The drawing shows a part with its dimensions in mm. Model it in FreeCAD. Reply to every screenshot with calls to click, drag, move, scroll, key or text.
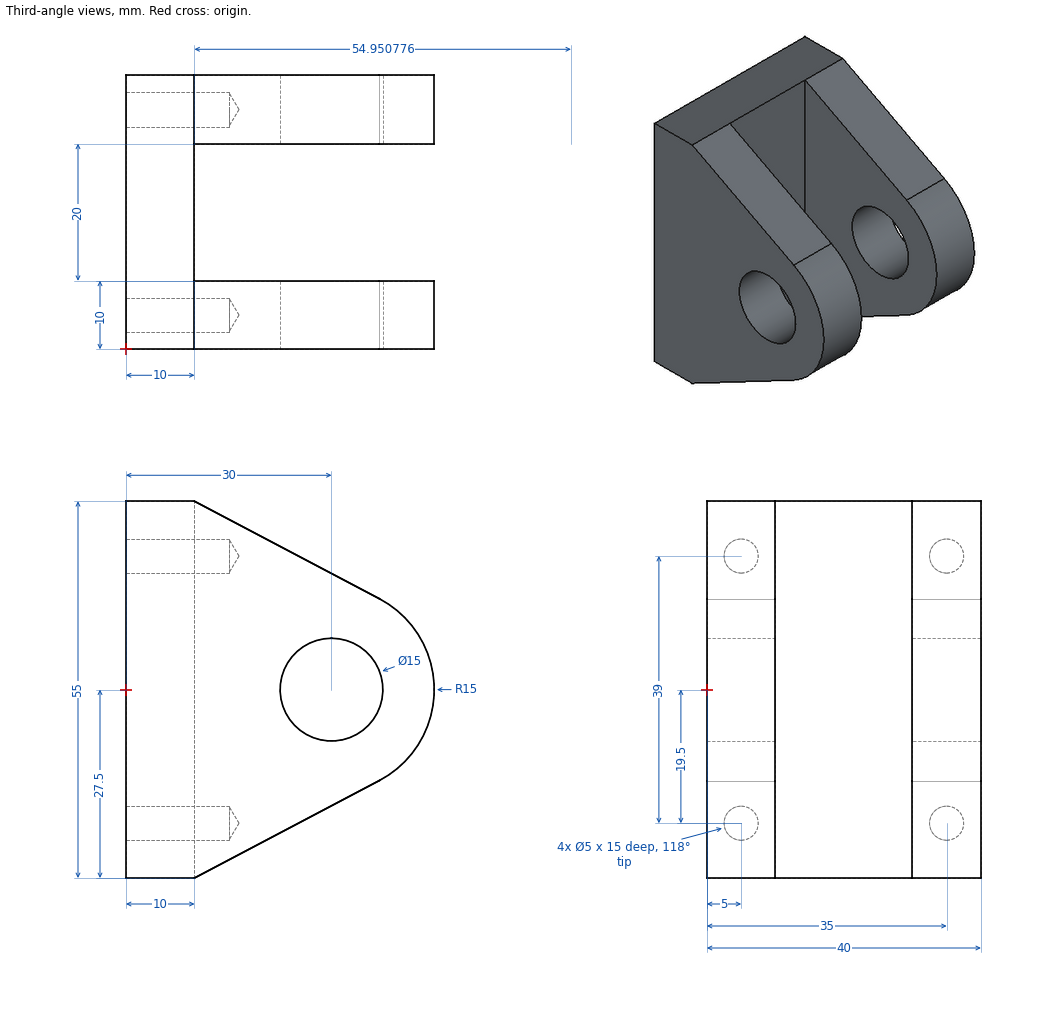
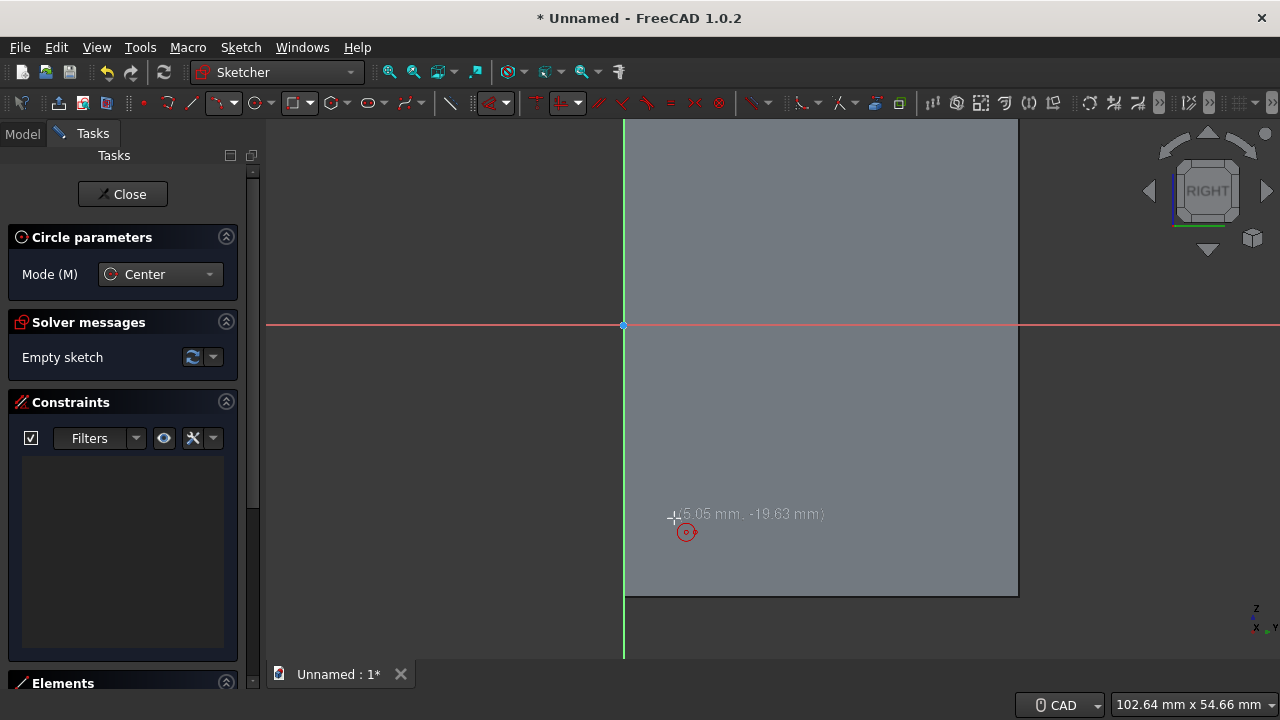
click(673, 518)
click(691, 500)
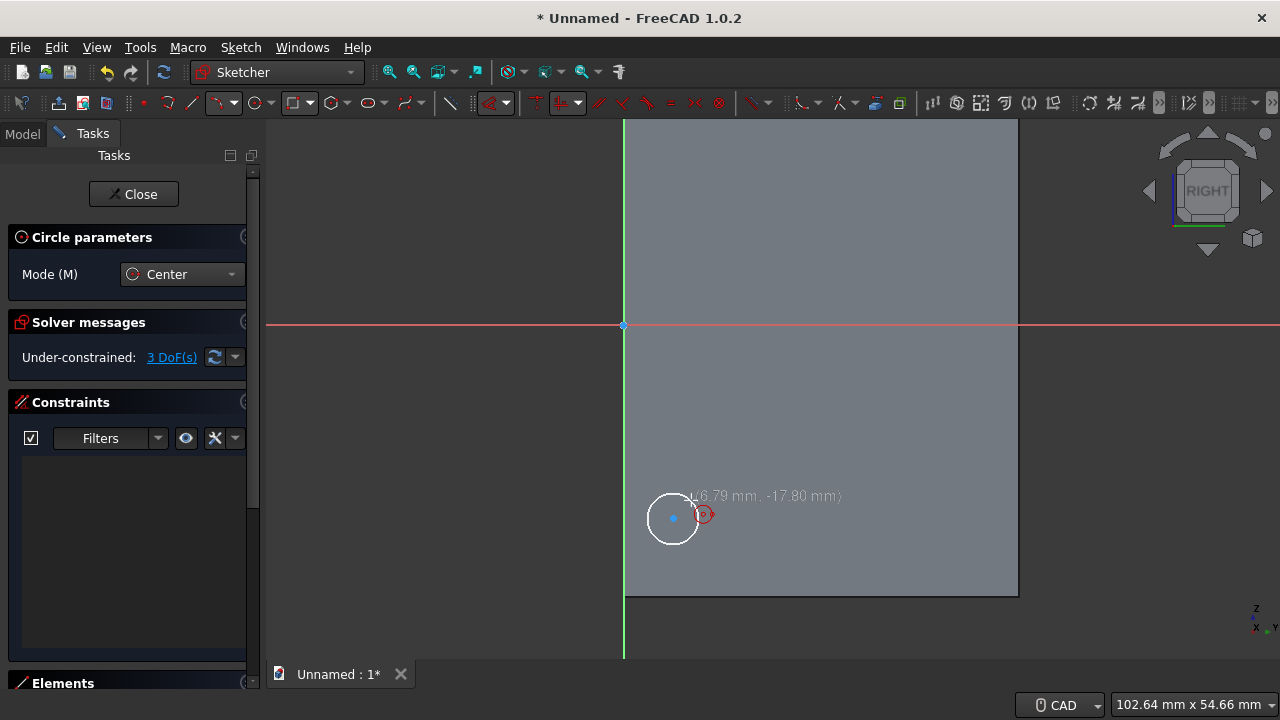
click(970, 518)
click(987, 500)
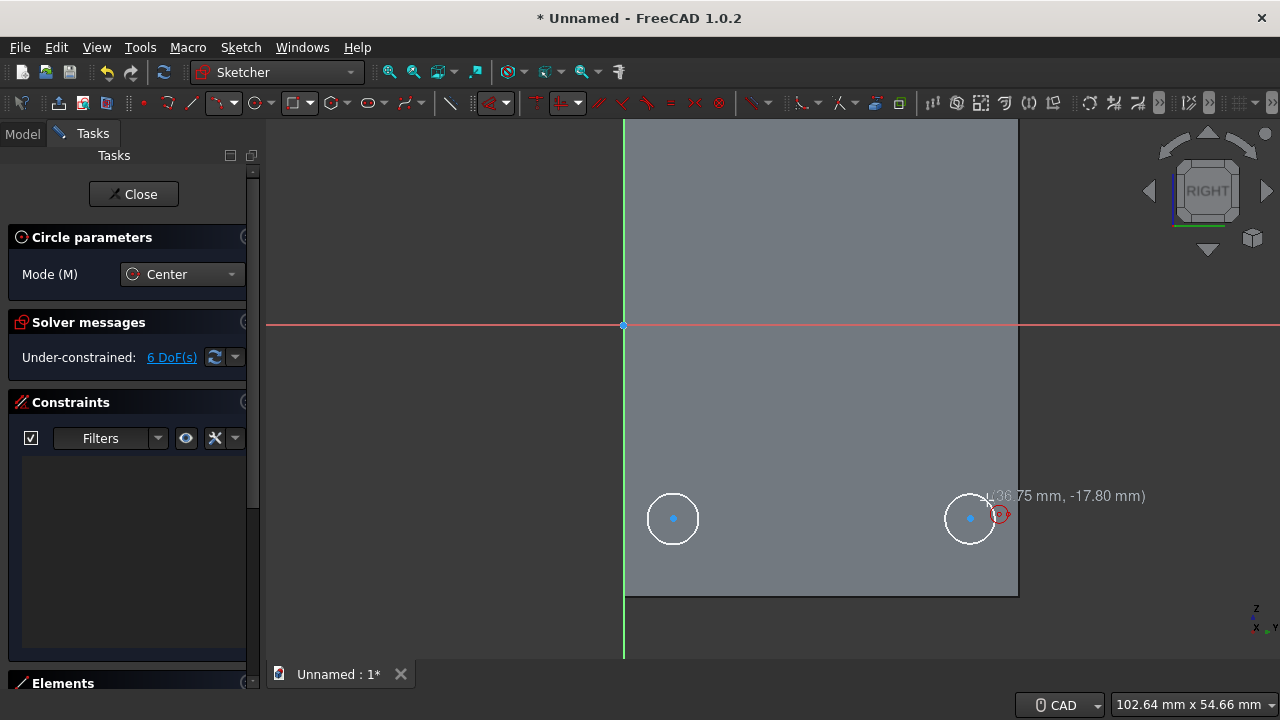
scroll(294, 631, down, 1)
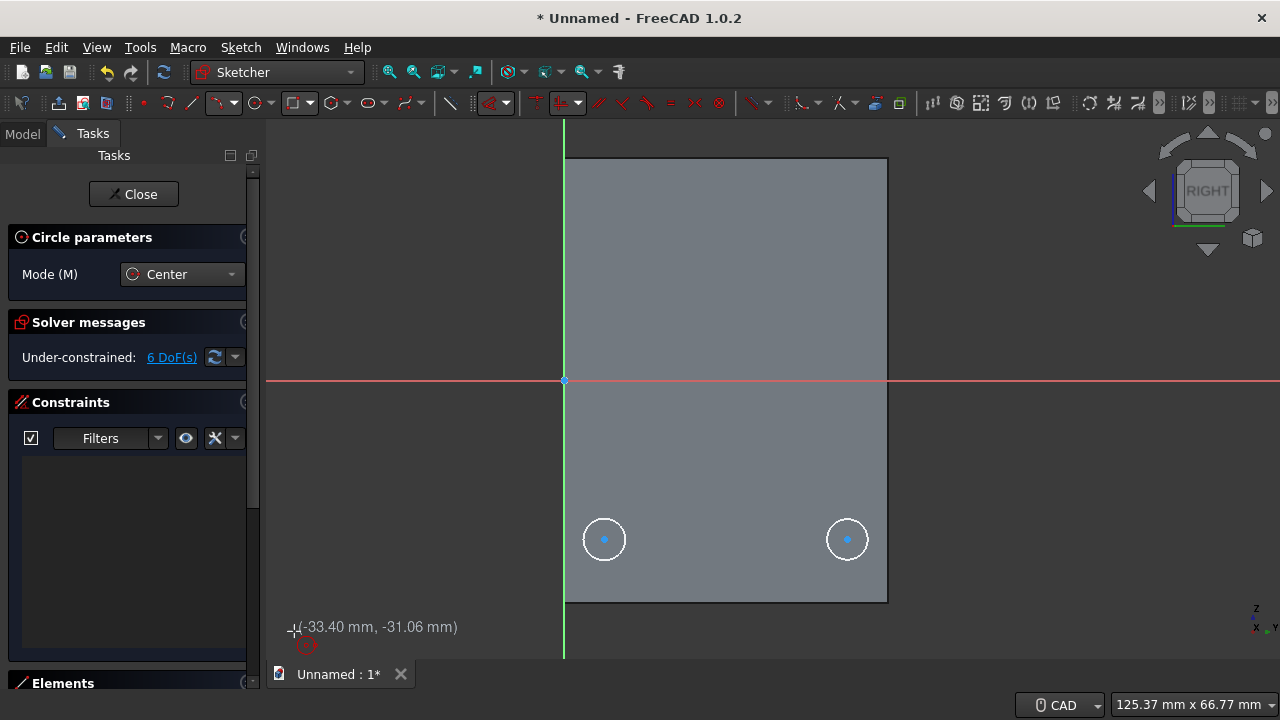
click(605, 223)
click(619, 209)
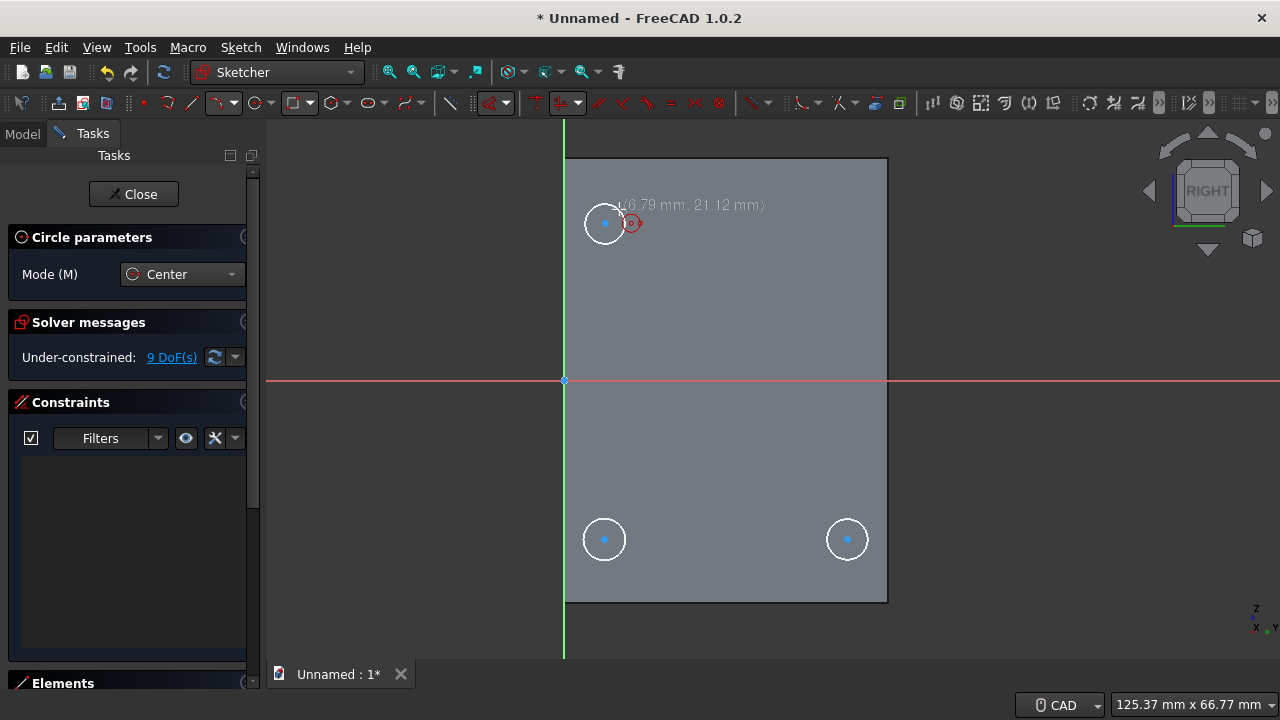
click(847, 223)
click(861, 209)
key(Escape)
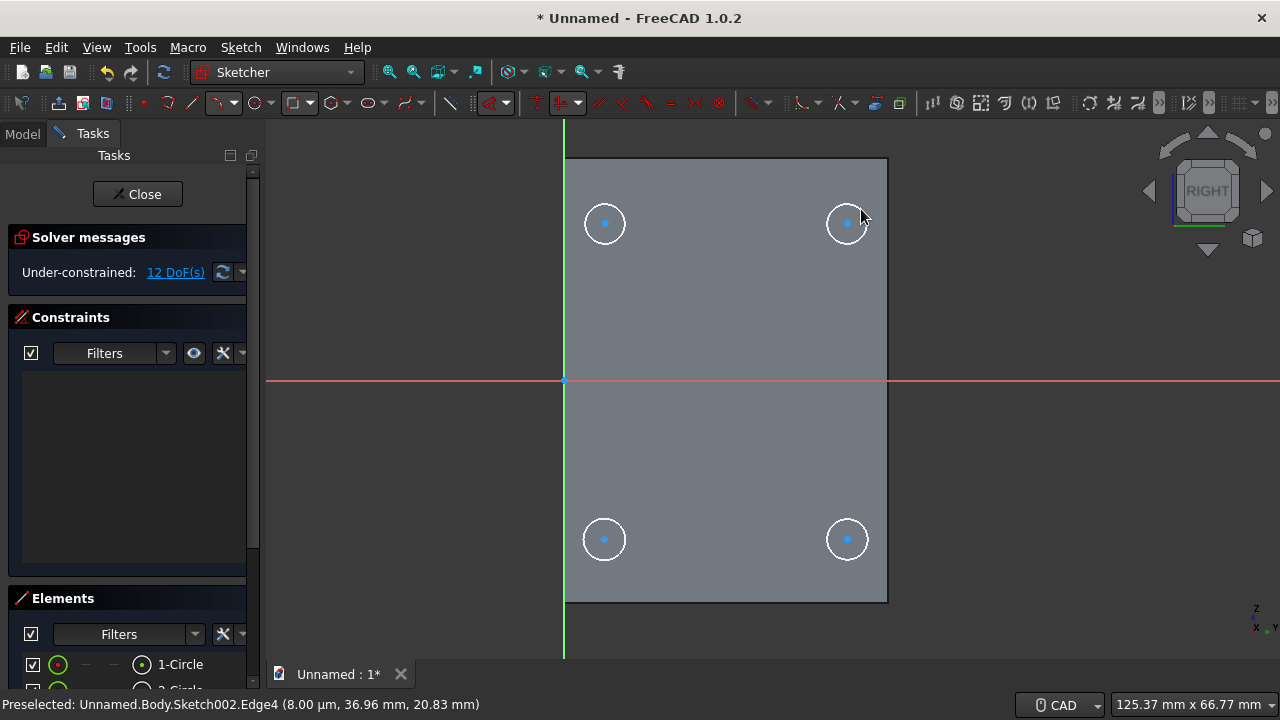
click(619, 525)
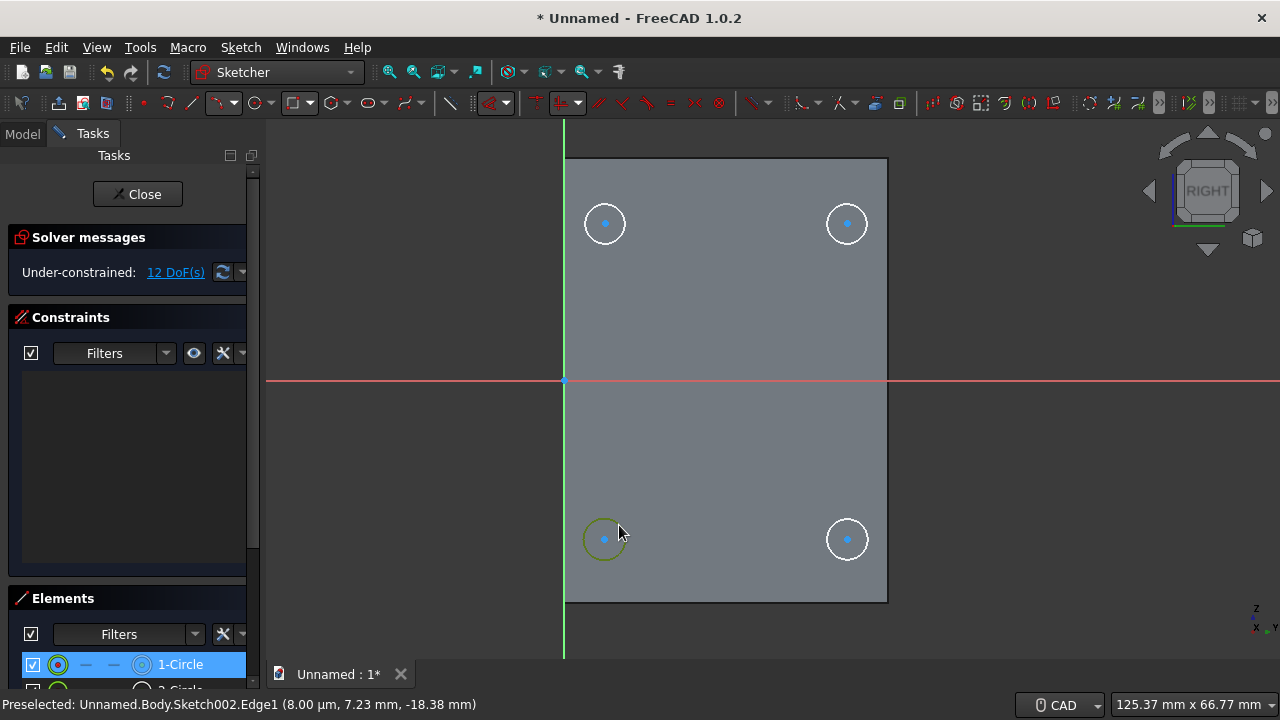
click(862, 525)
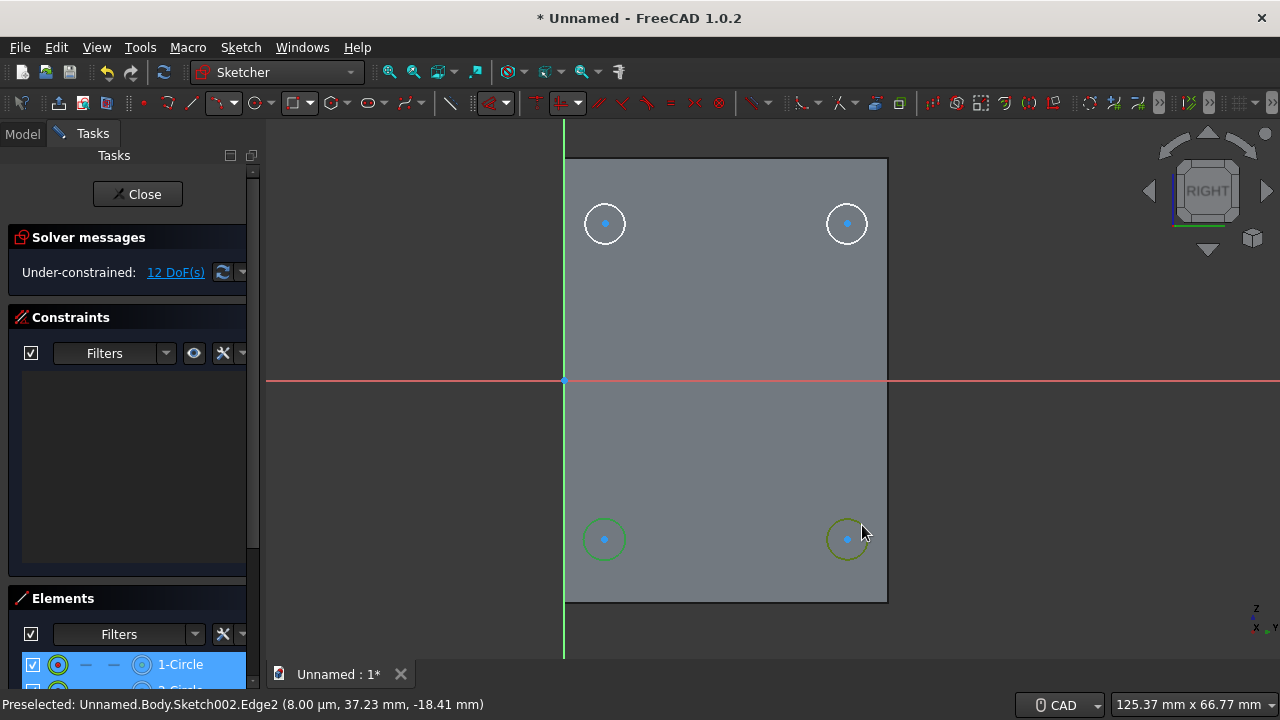
click(619, 210)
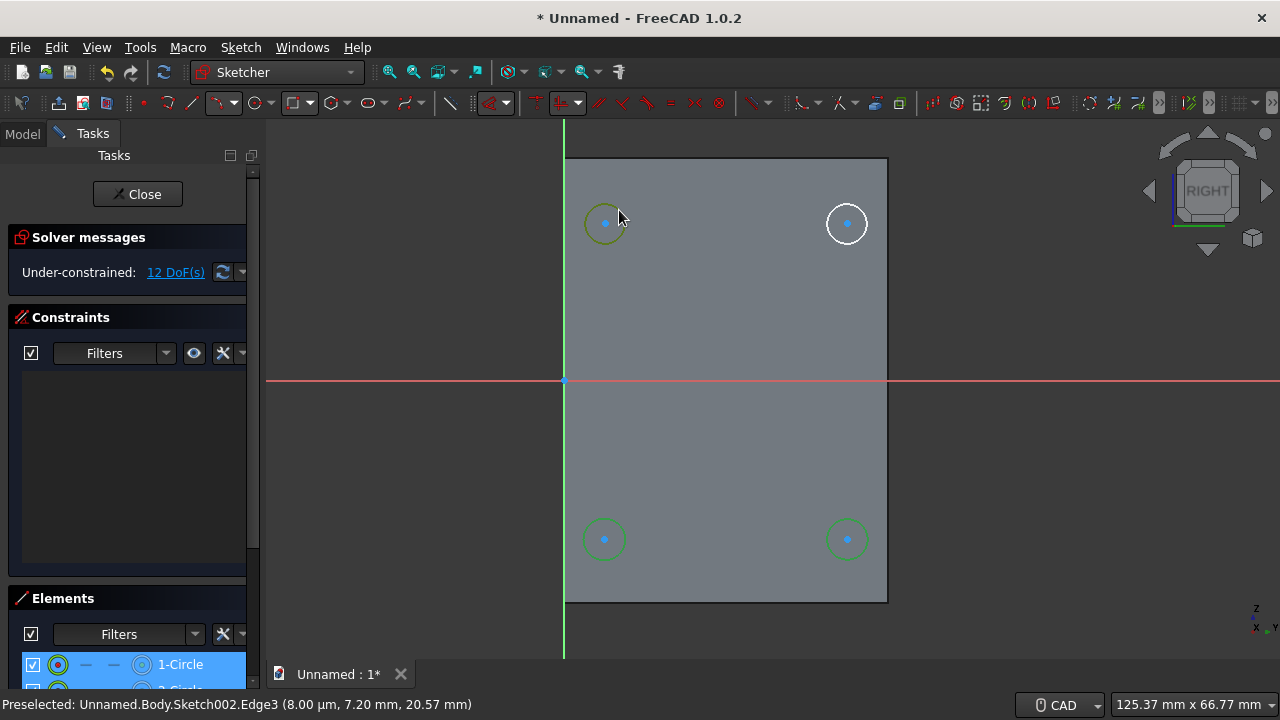
click(861, 210)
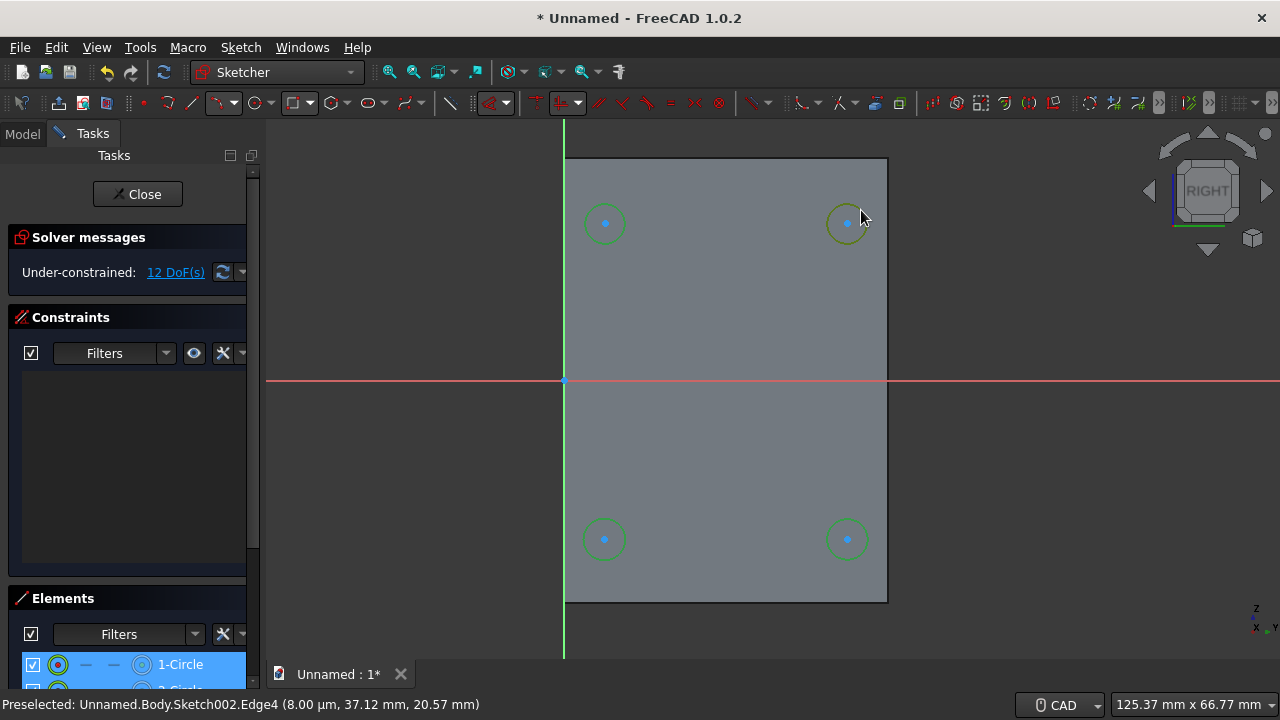
key(e)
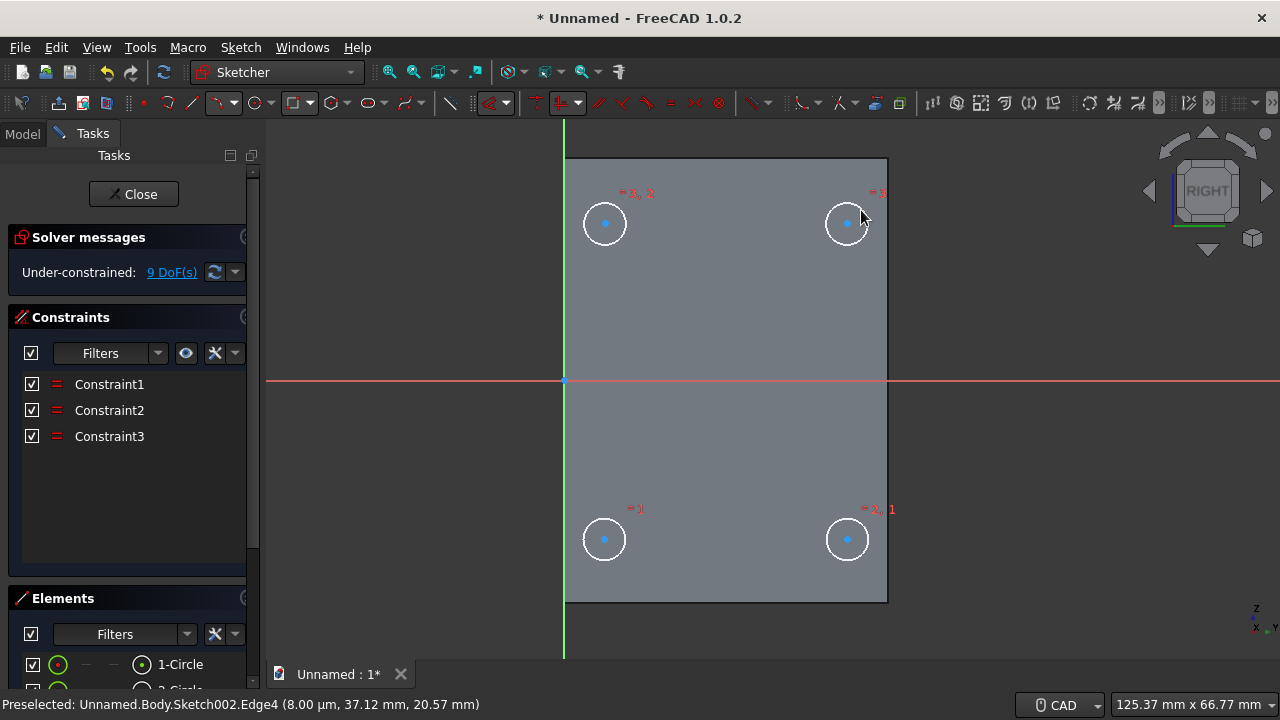
click(619, 525)